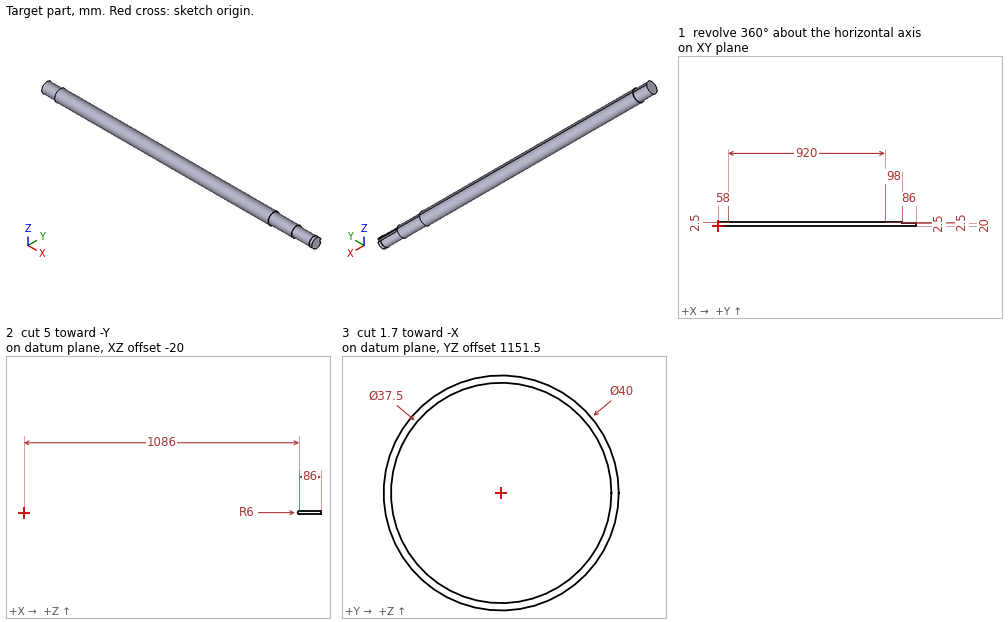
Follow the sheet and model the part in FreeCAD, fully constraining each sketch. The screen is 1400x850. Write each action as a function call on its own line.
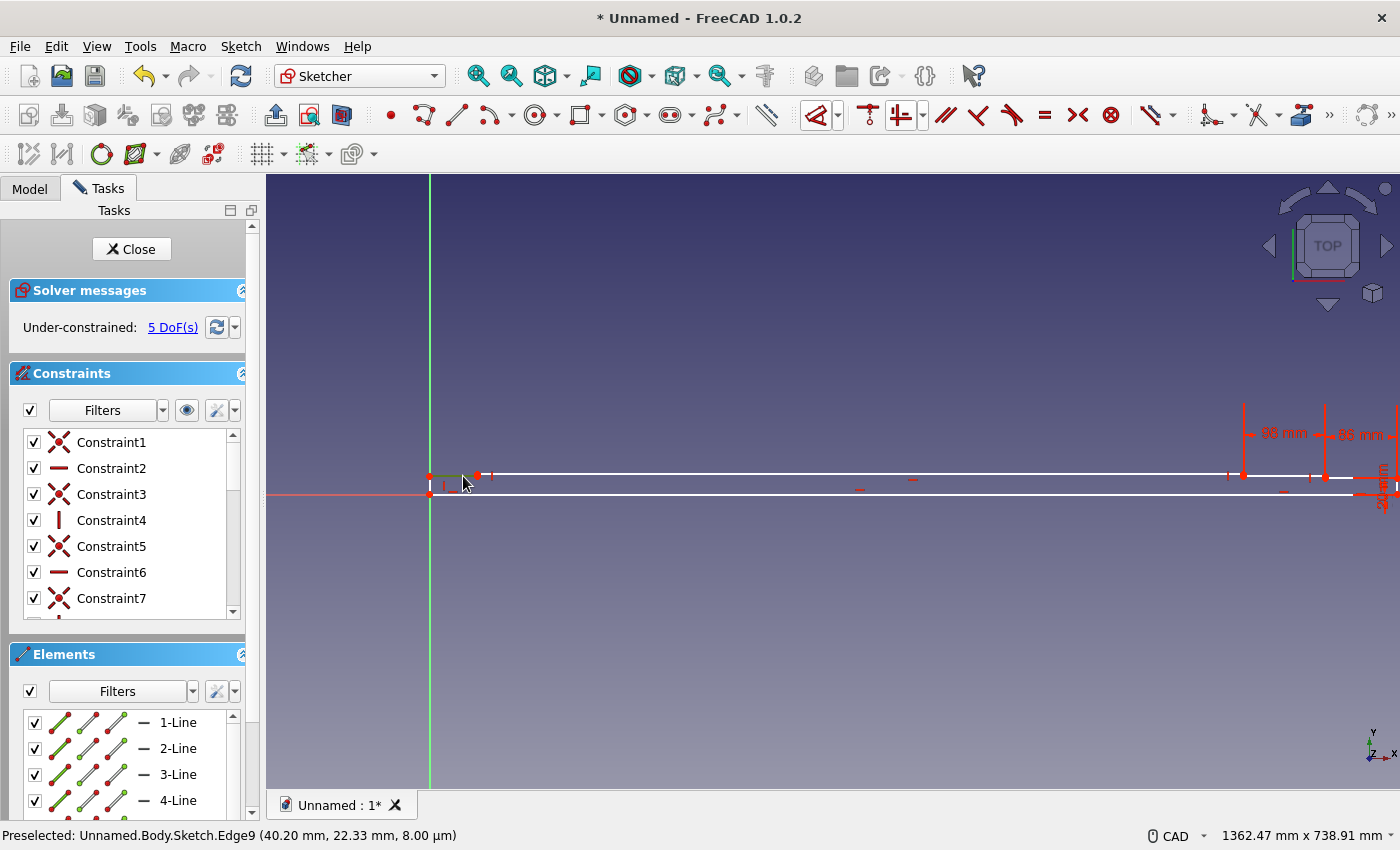
click(838, 116)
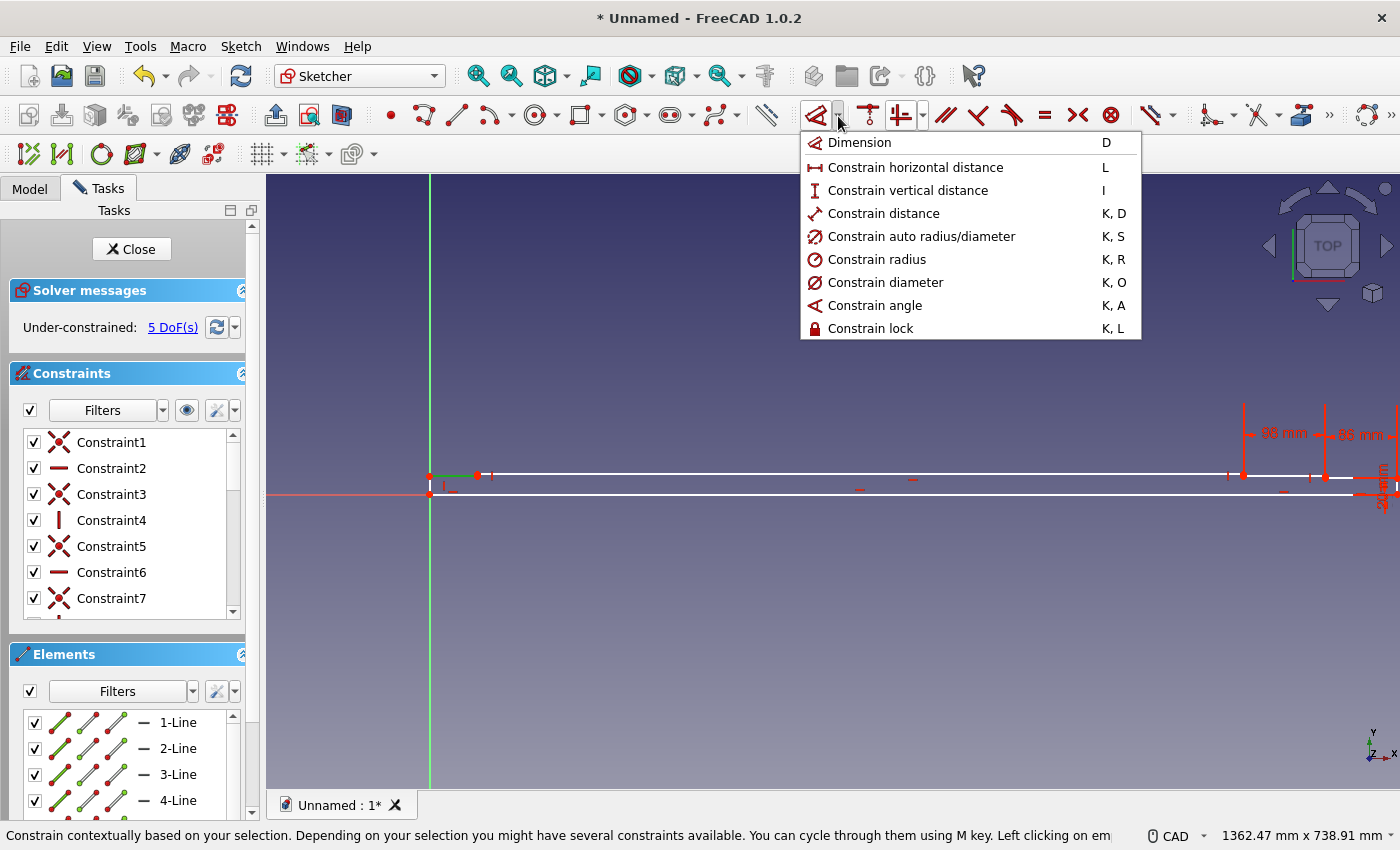
click(971, 168)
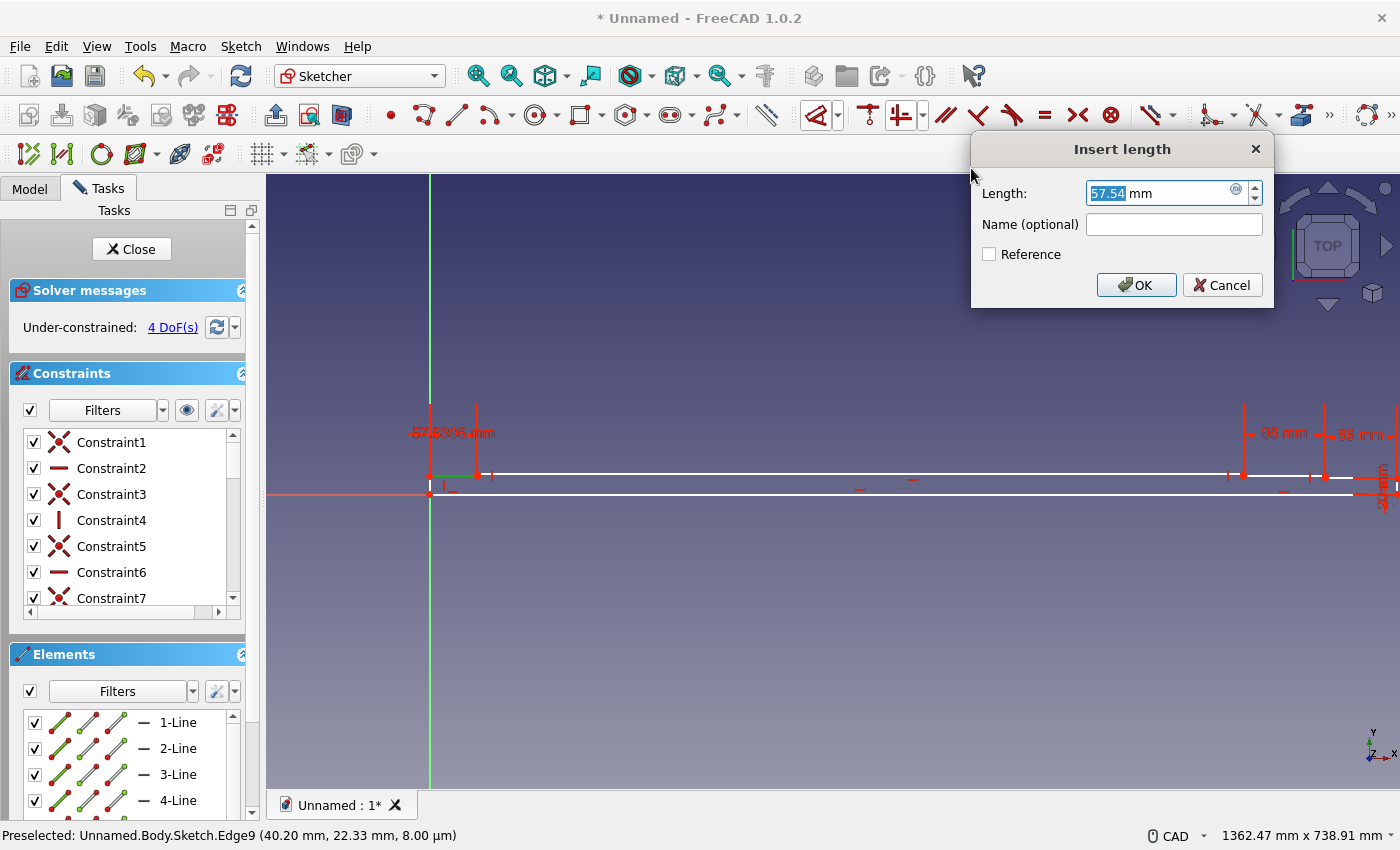
text(58)
key(Return)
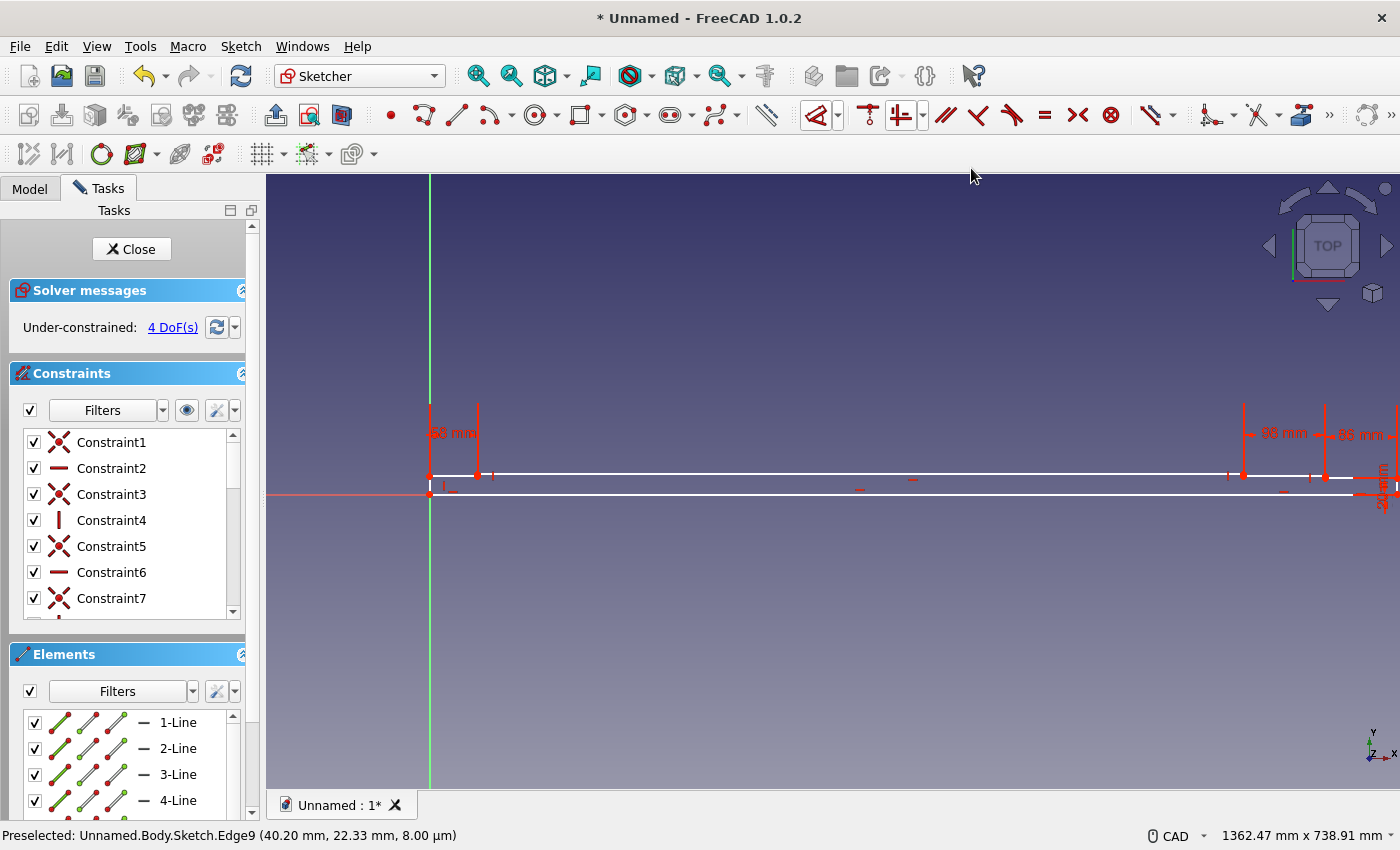
scroll(462, 476, down, 2)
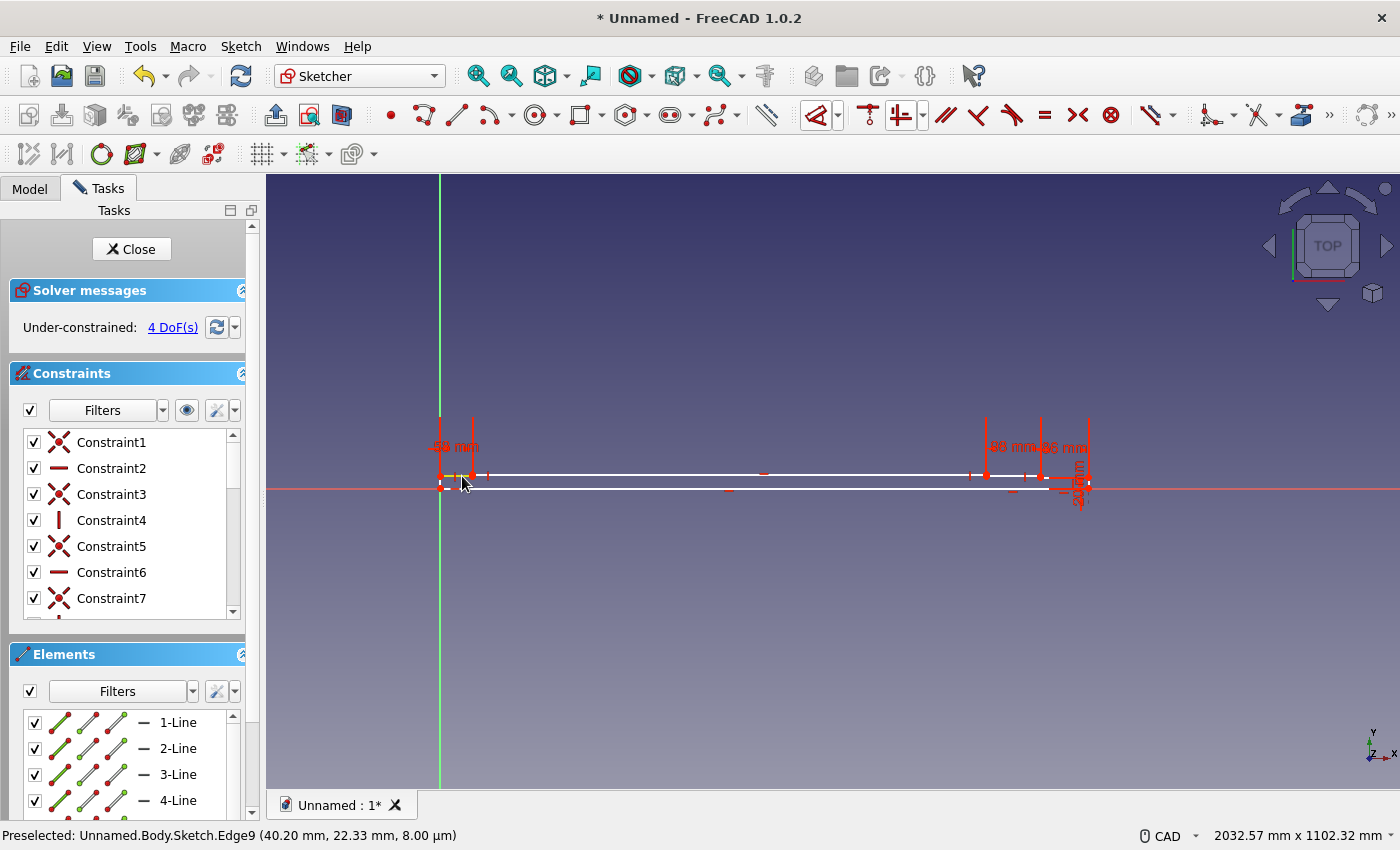
scroll(1041, 477, up, 17)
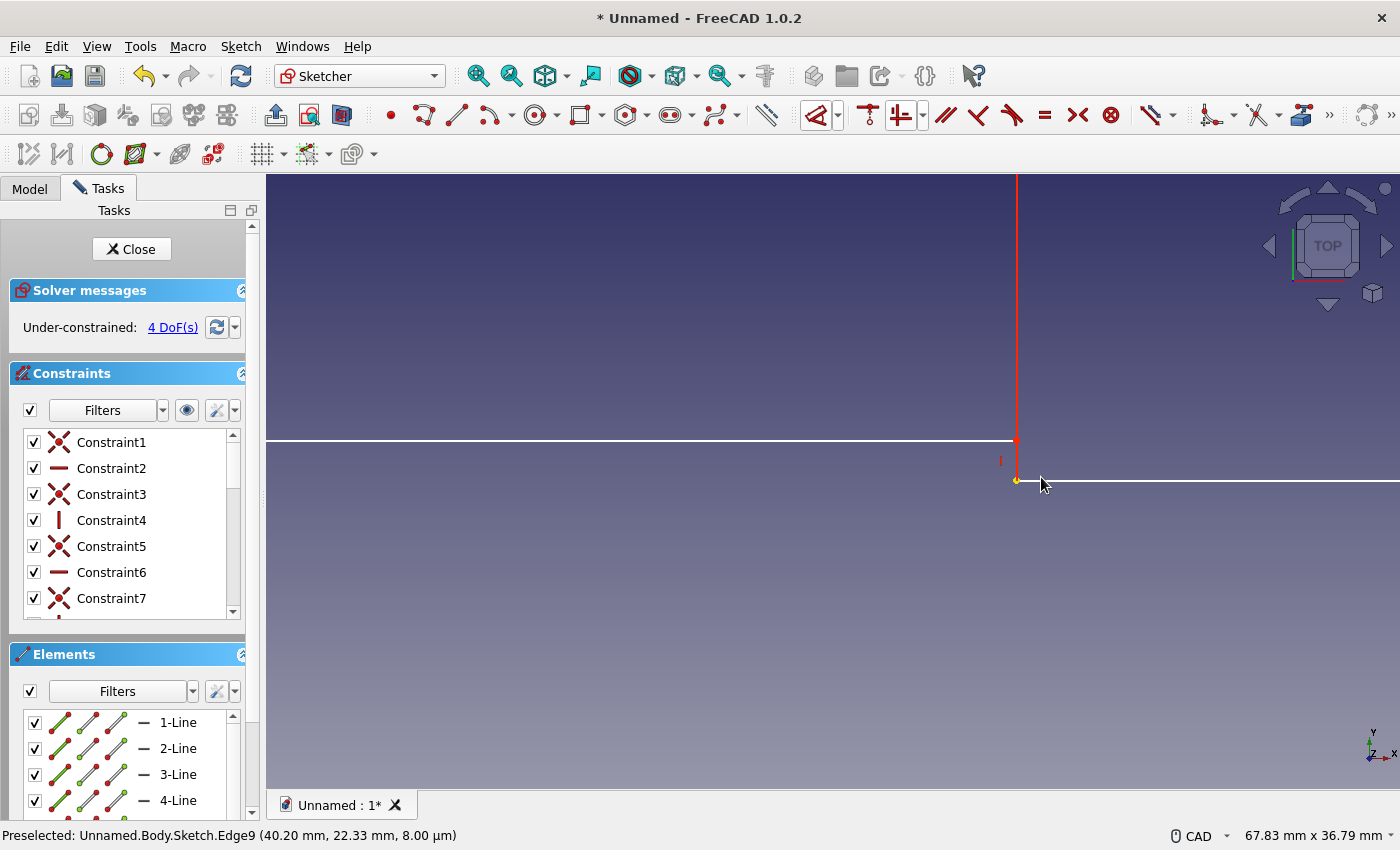
click(1017, 461)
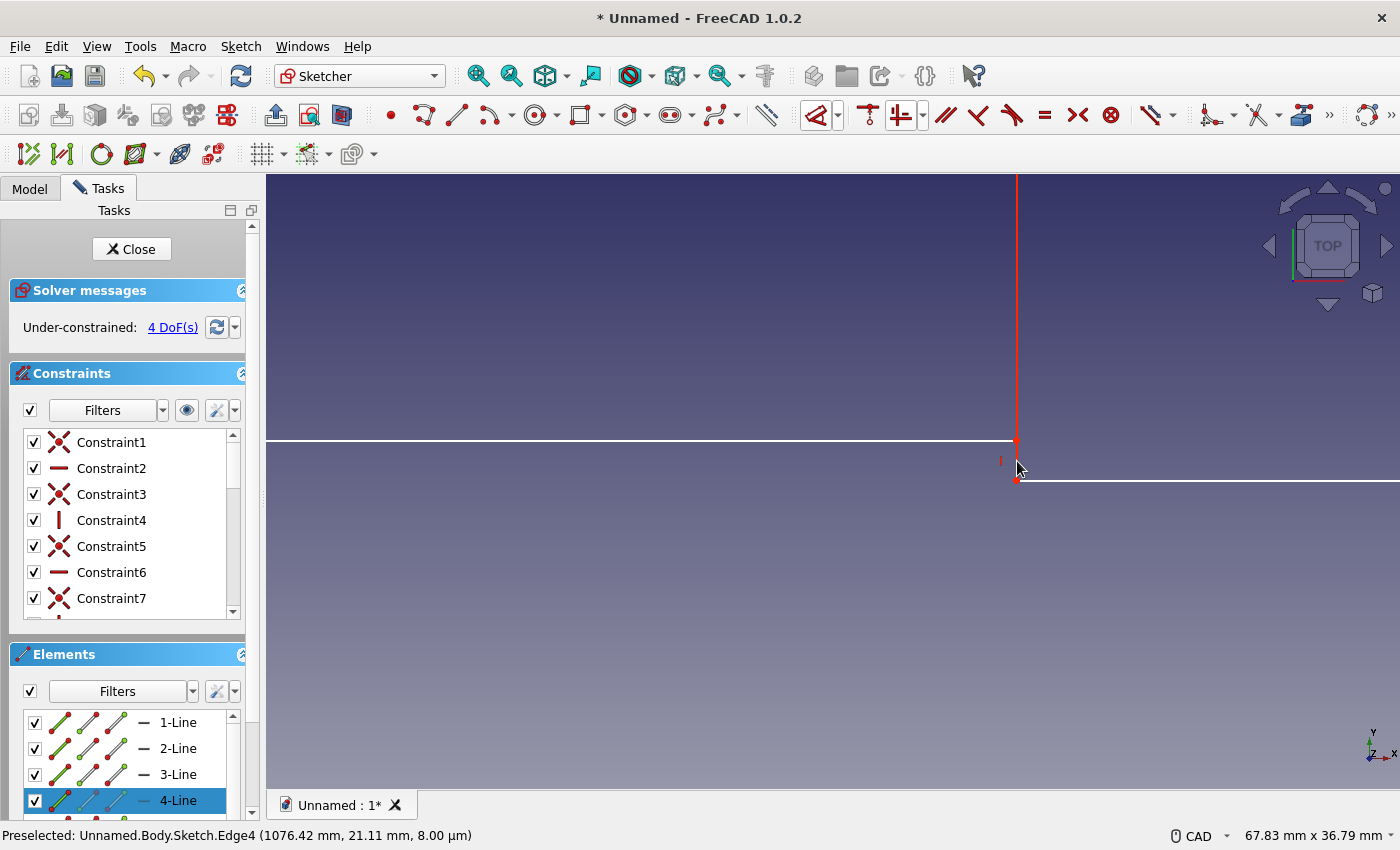
click(838, 116)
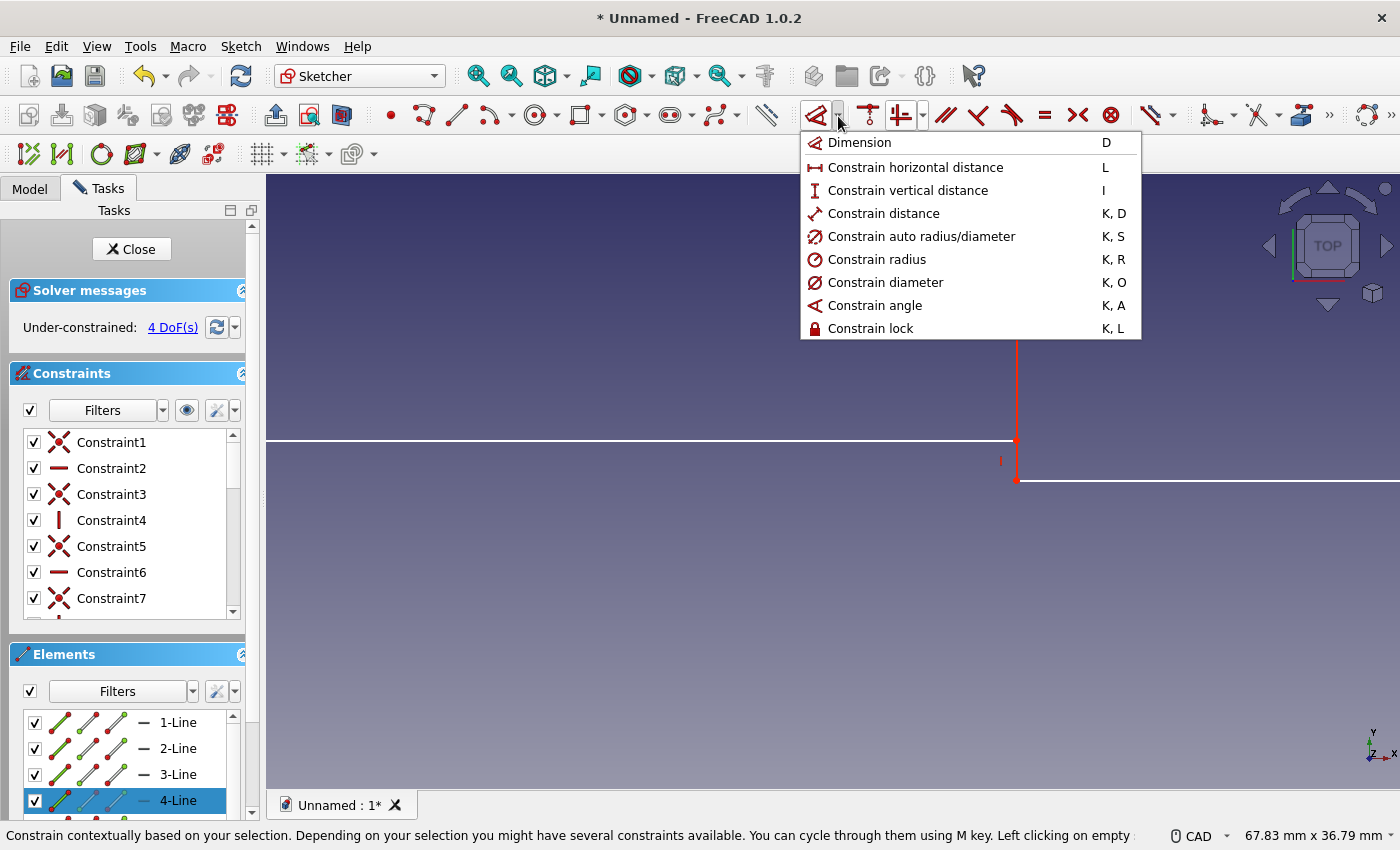
click(971, 190)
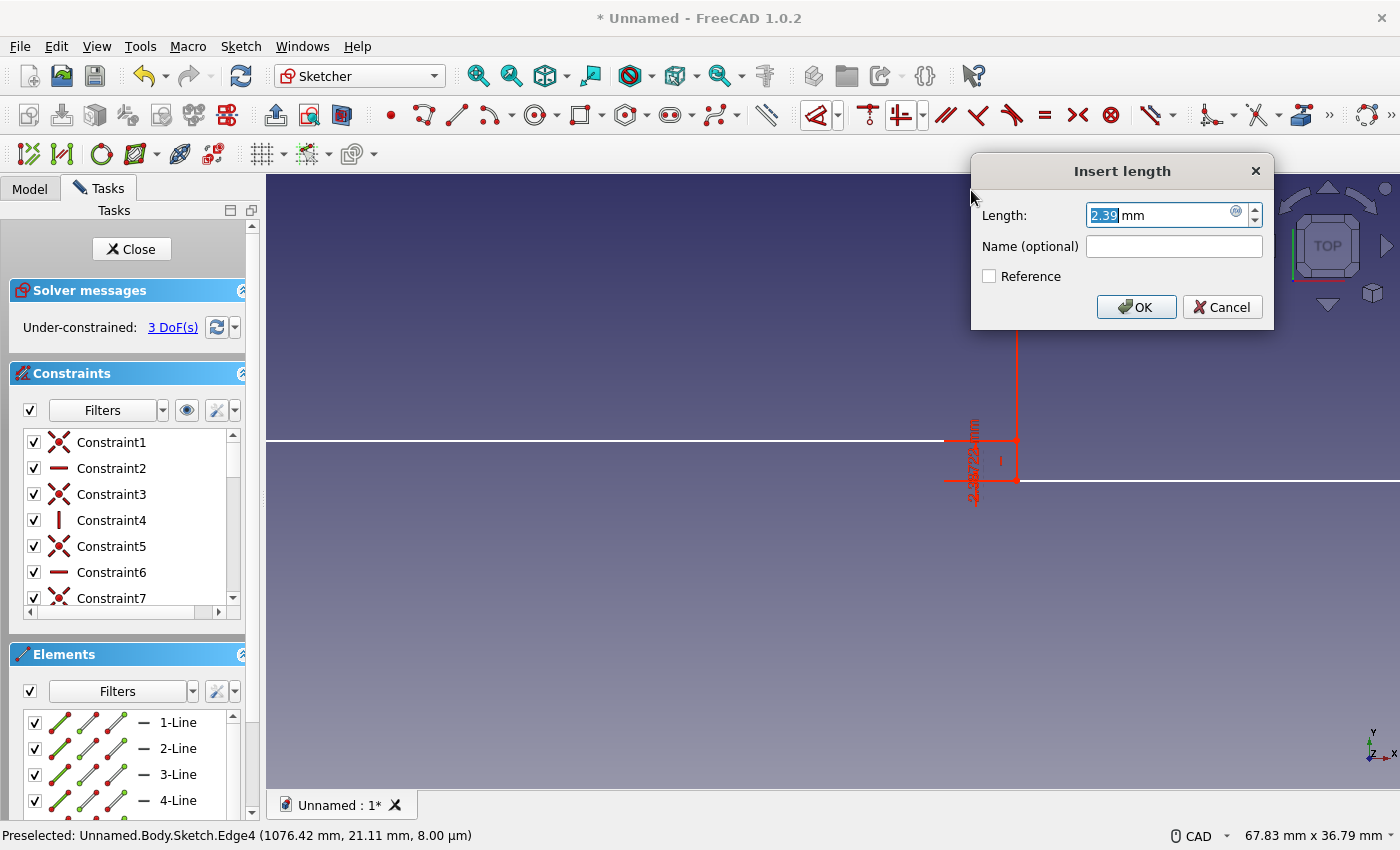
text(2.5)
key(Return)